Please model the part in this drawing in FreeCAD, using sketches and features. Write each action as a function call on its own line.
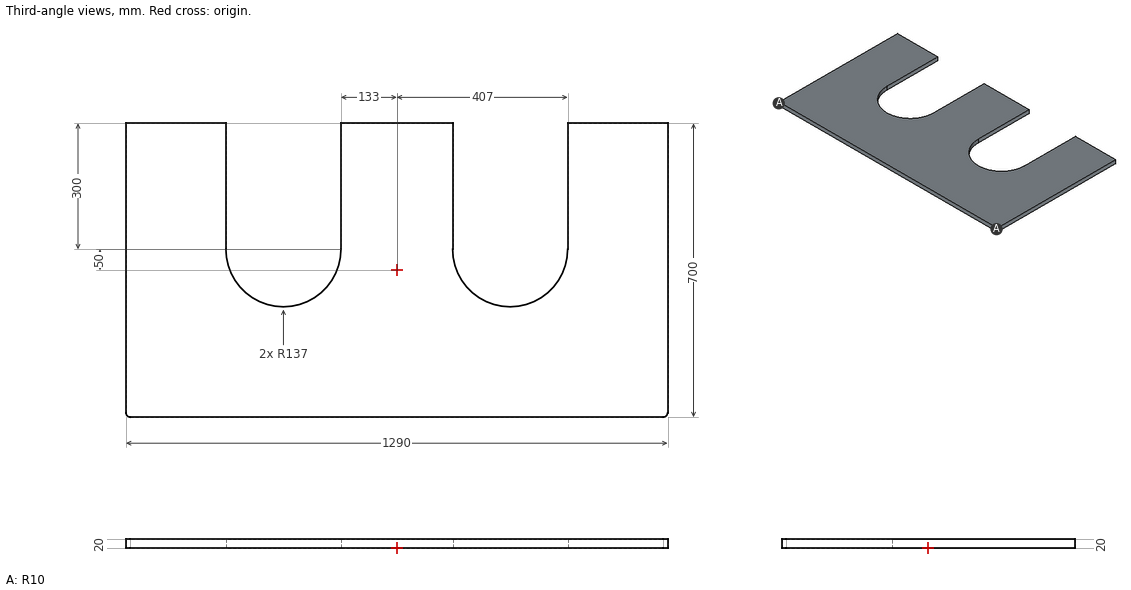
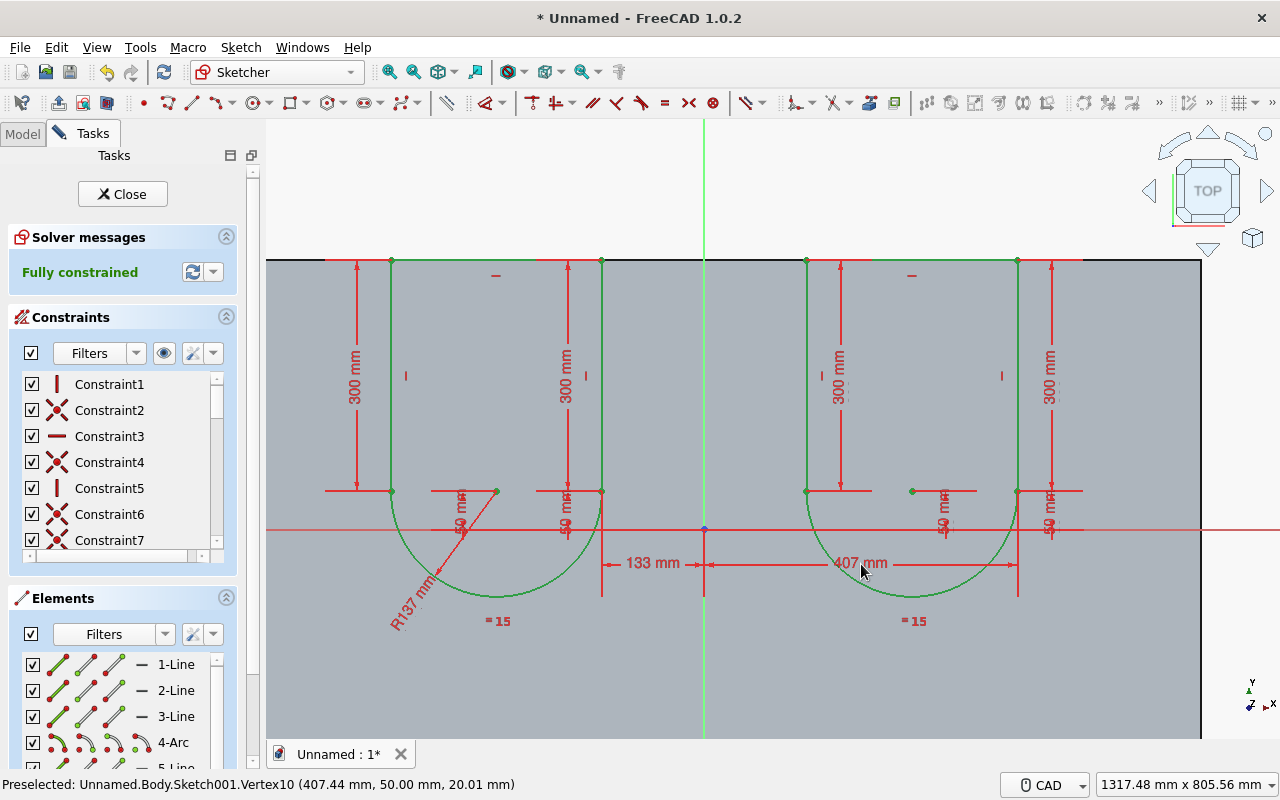
click(123, 194)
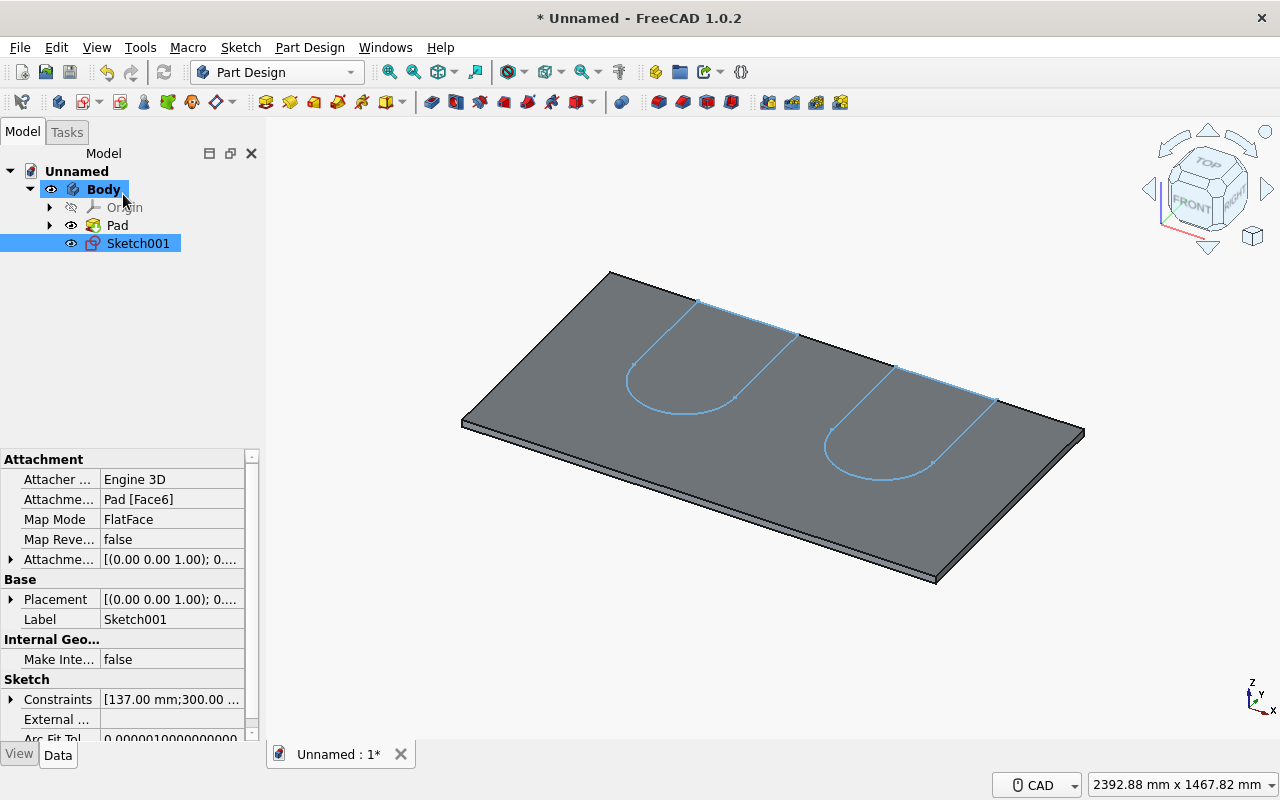
click(432, 102)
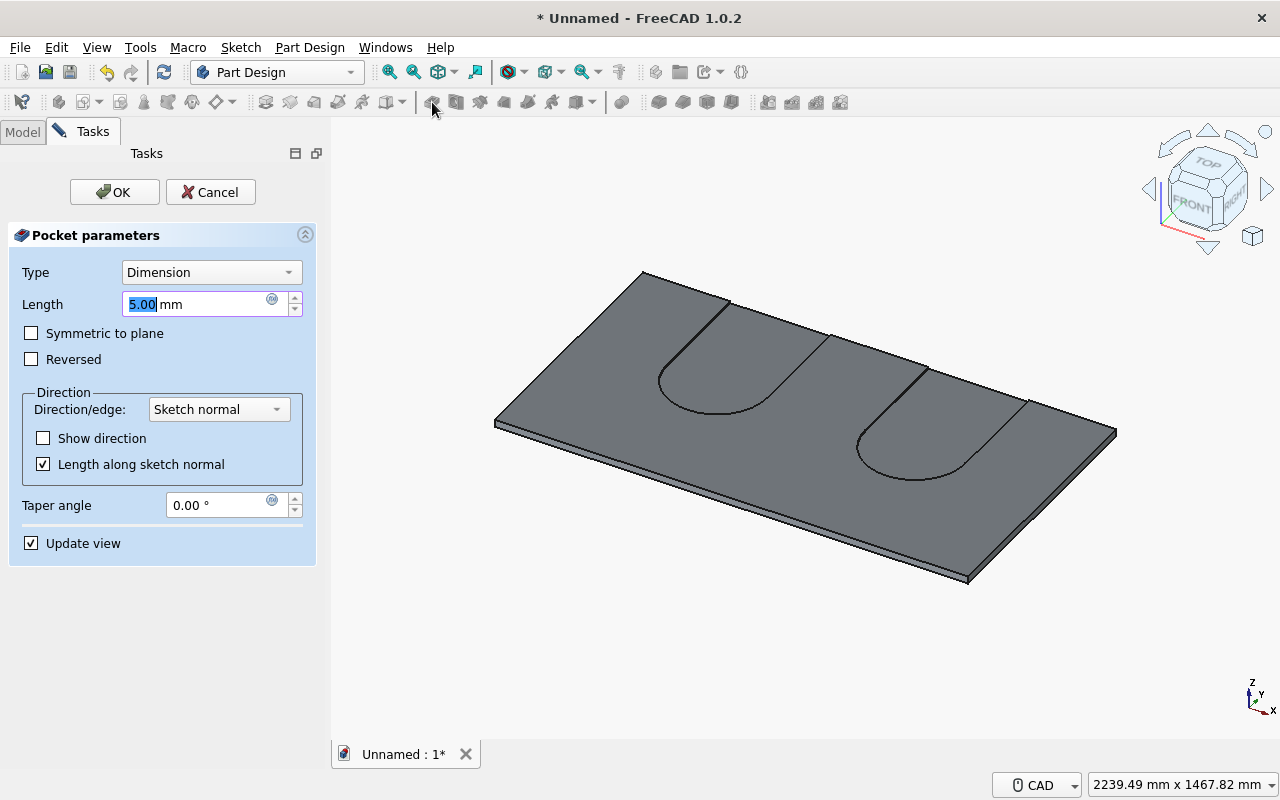
text(20)
key(Tab)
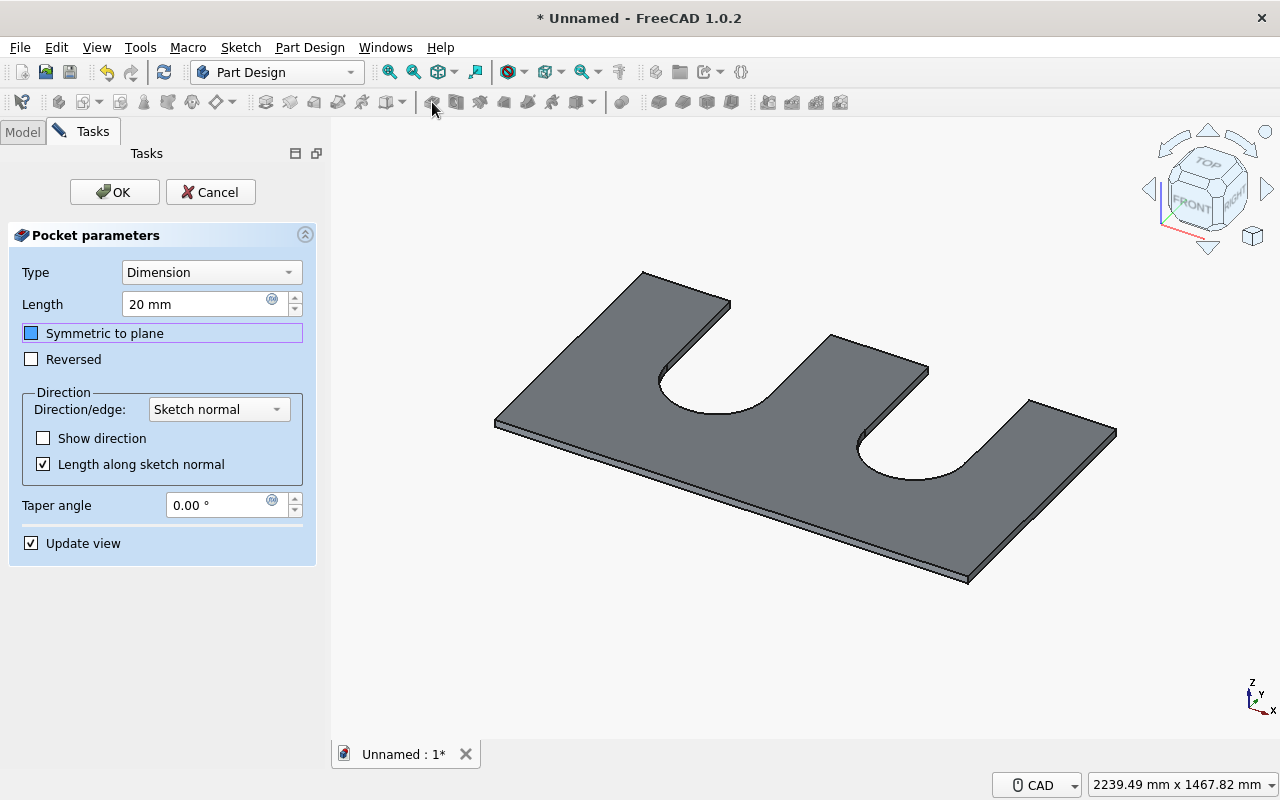
click(115, 192)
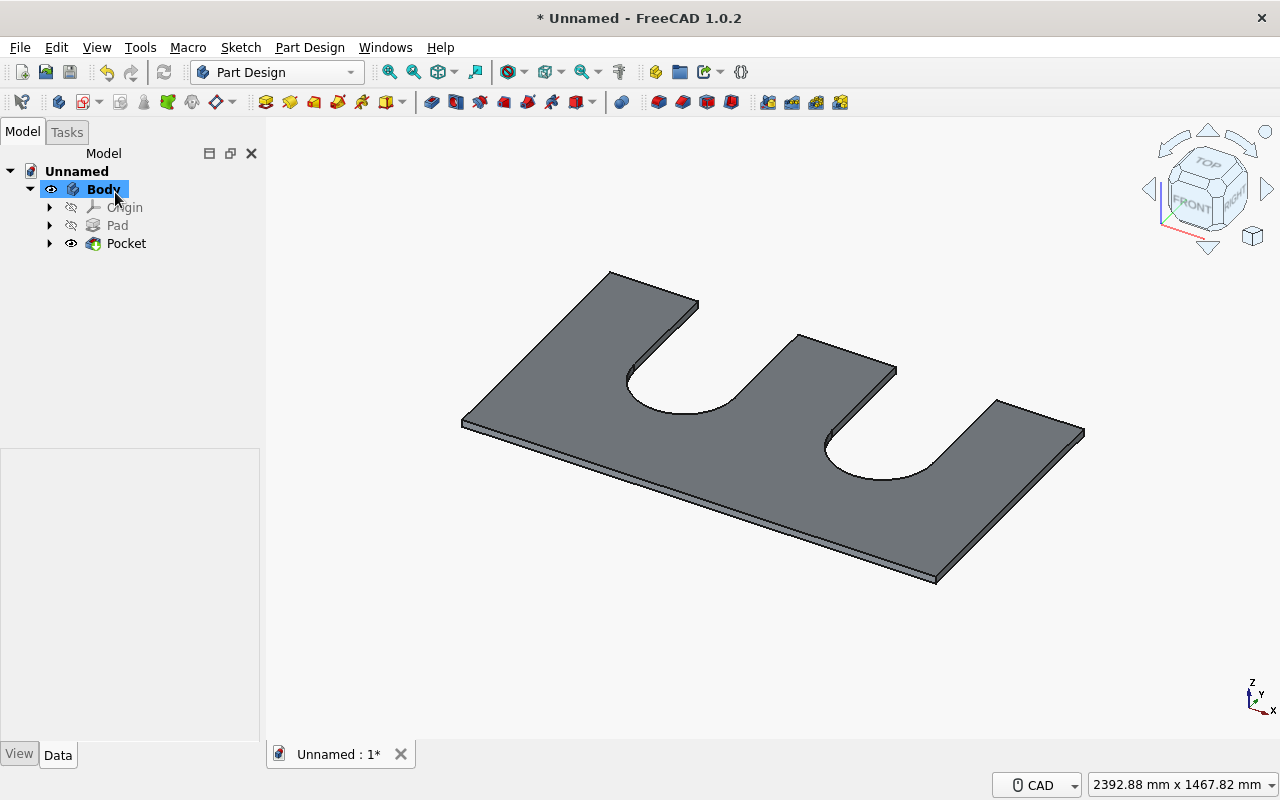
scroll(936, 579, up, 8)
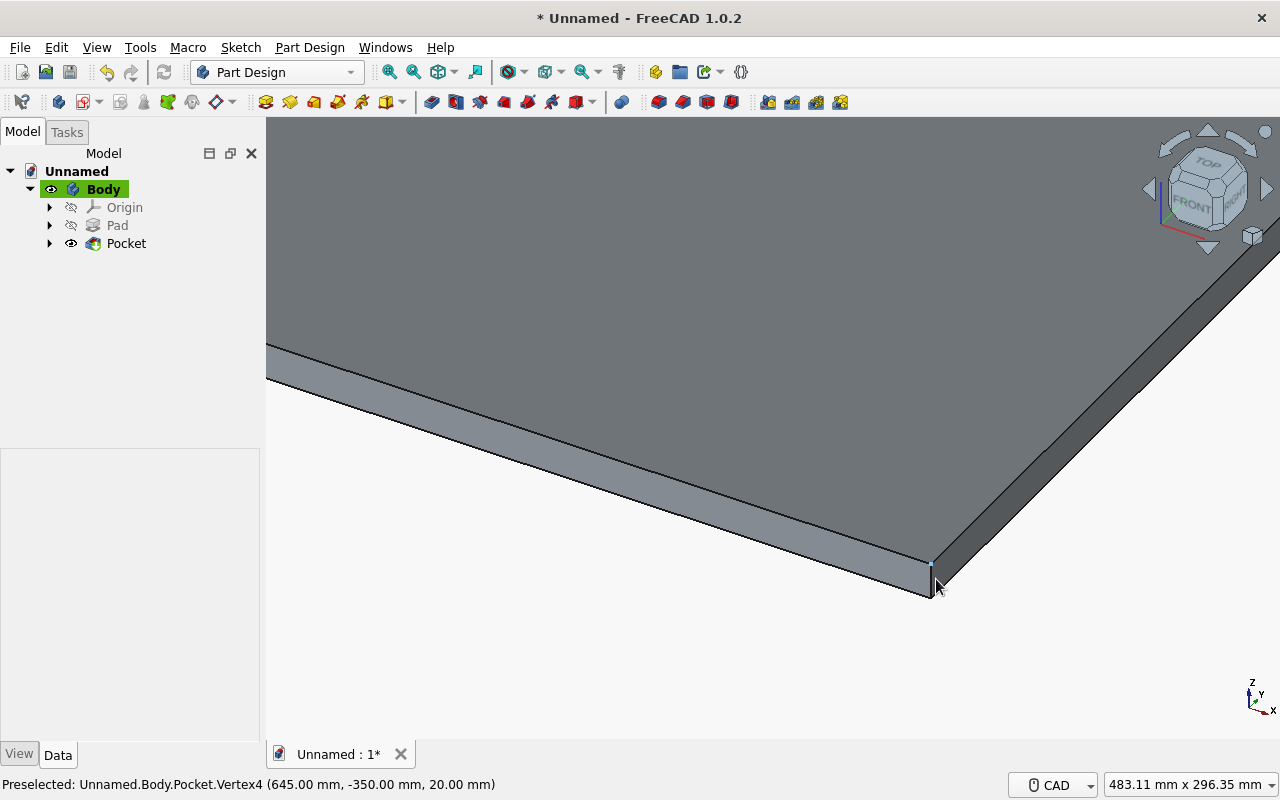
click(931, 580)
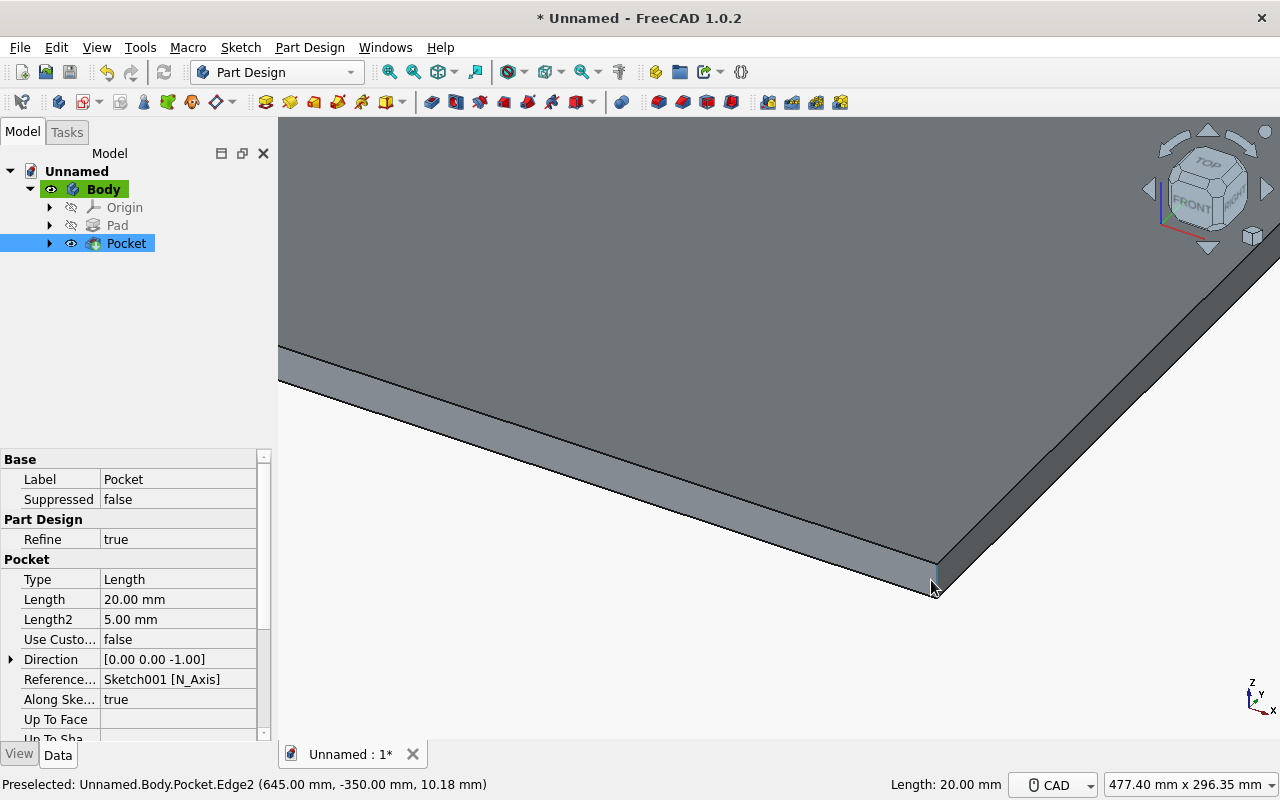
key(v)
key(f)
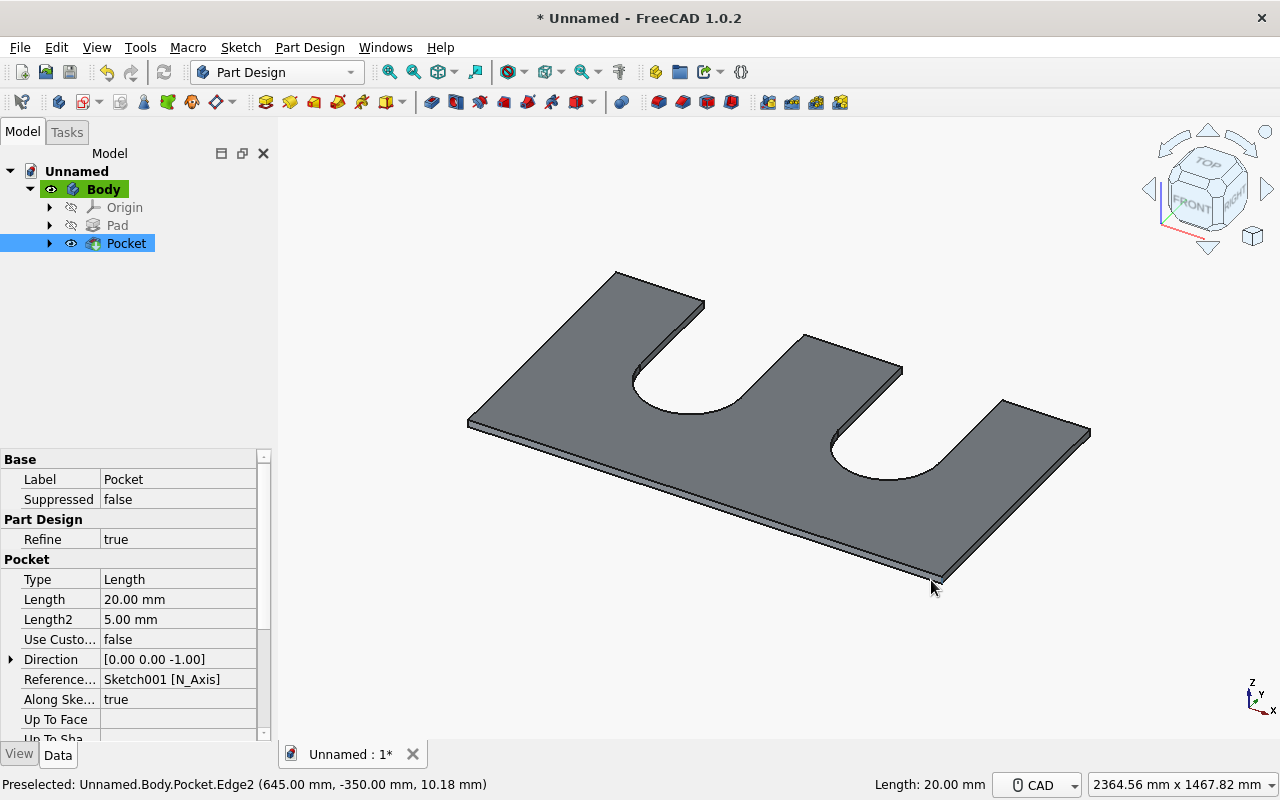
key(0)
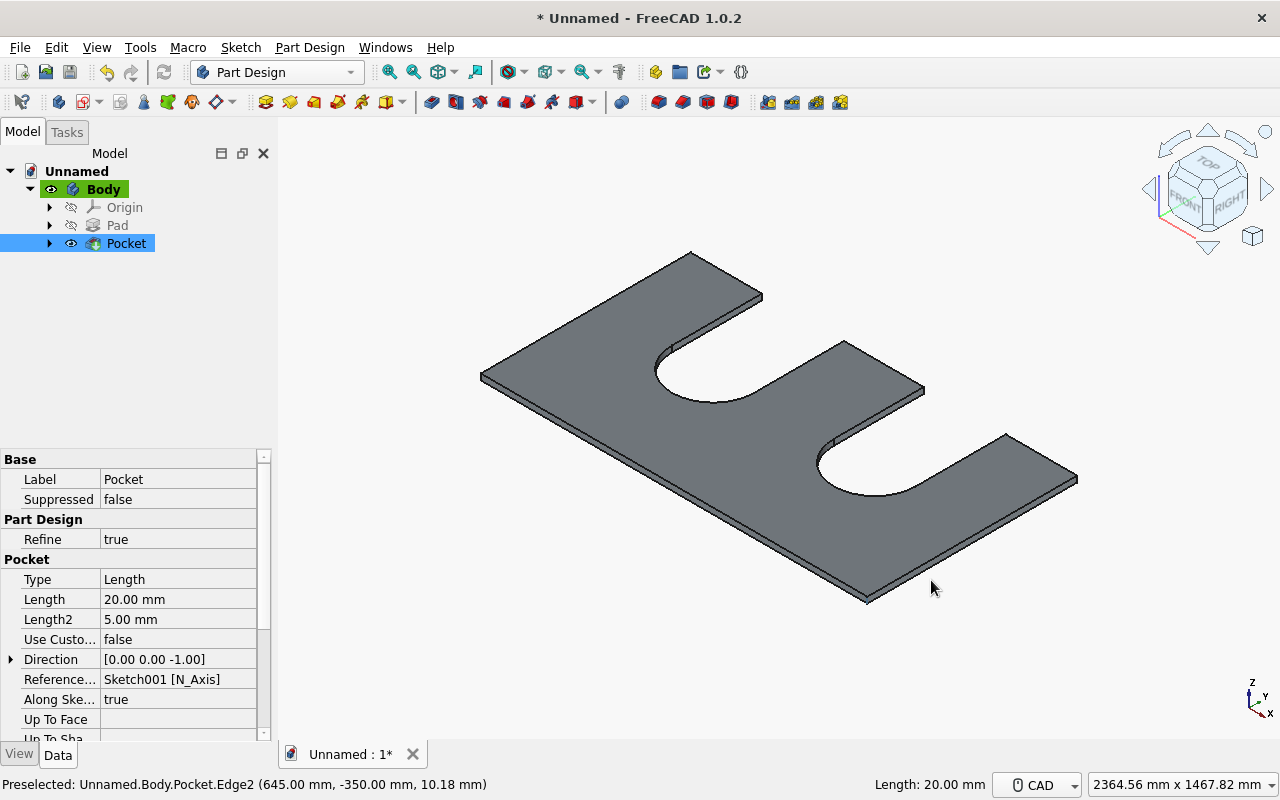
scroll(481, 376, up, 8)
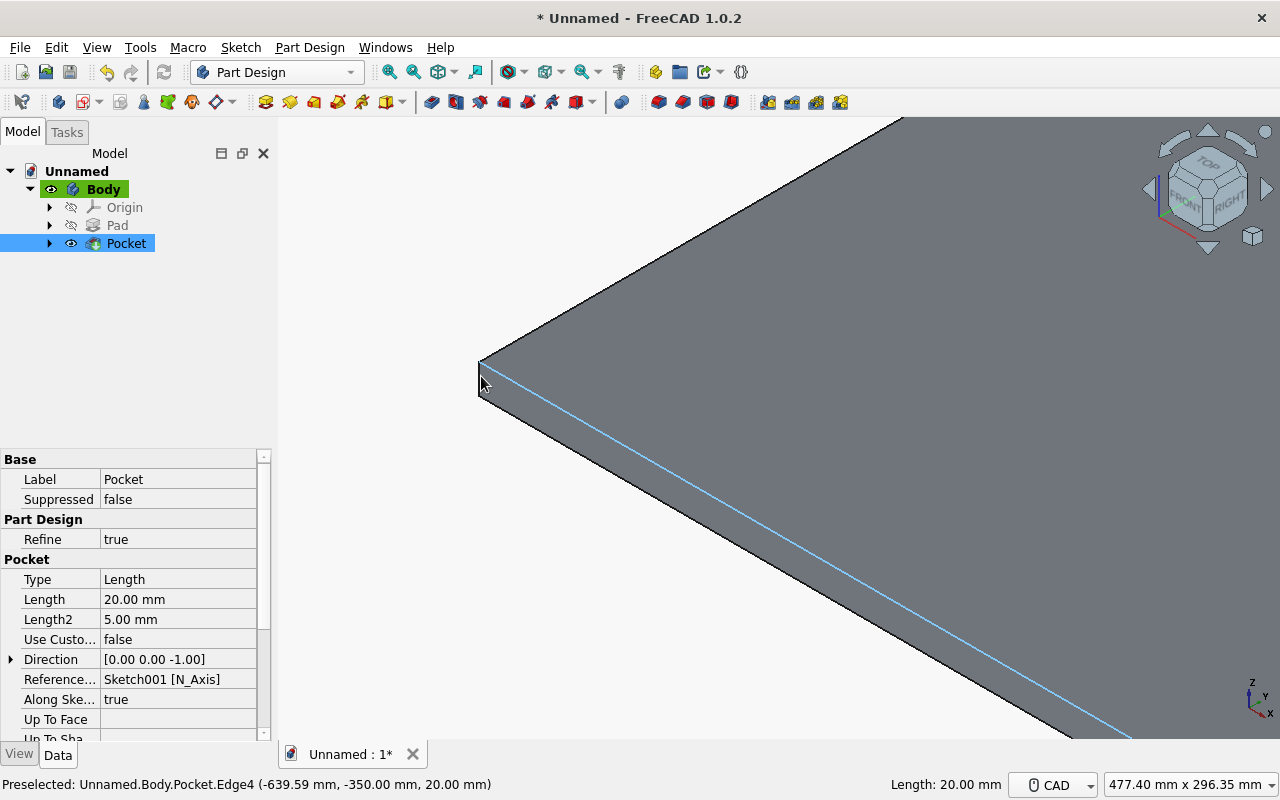
key(v)
key(f)